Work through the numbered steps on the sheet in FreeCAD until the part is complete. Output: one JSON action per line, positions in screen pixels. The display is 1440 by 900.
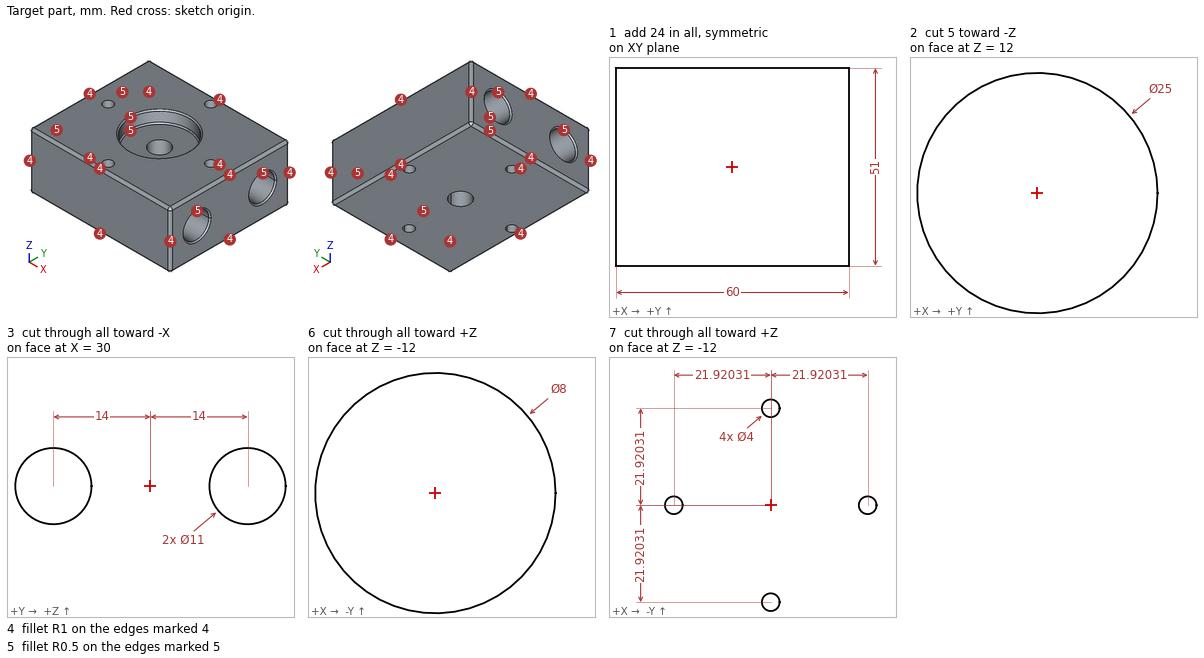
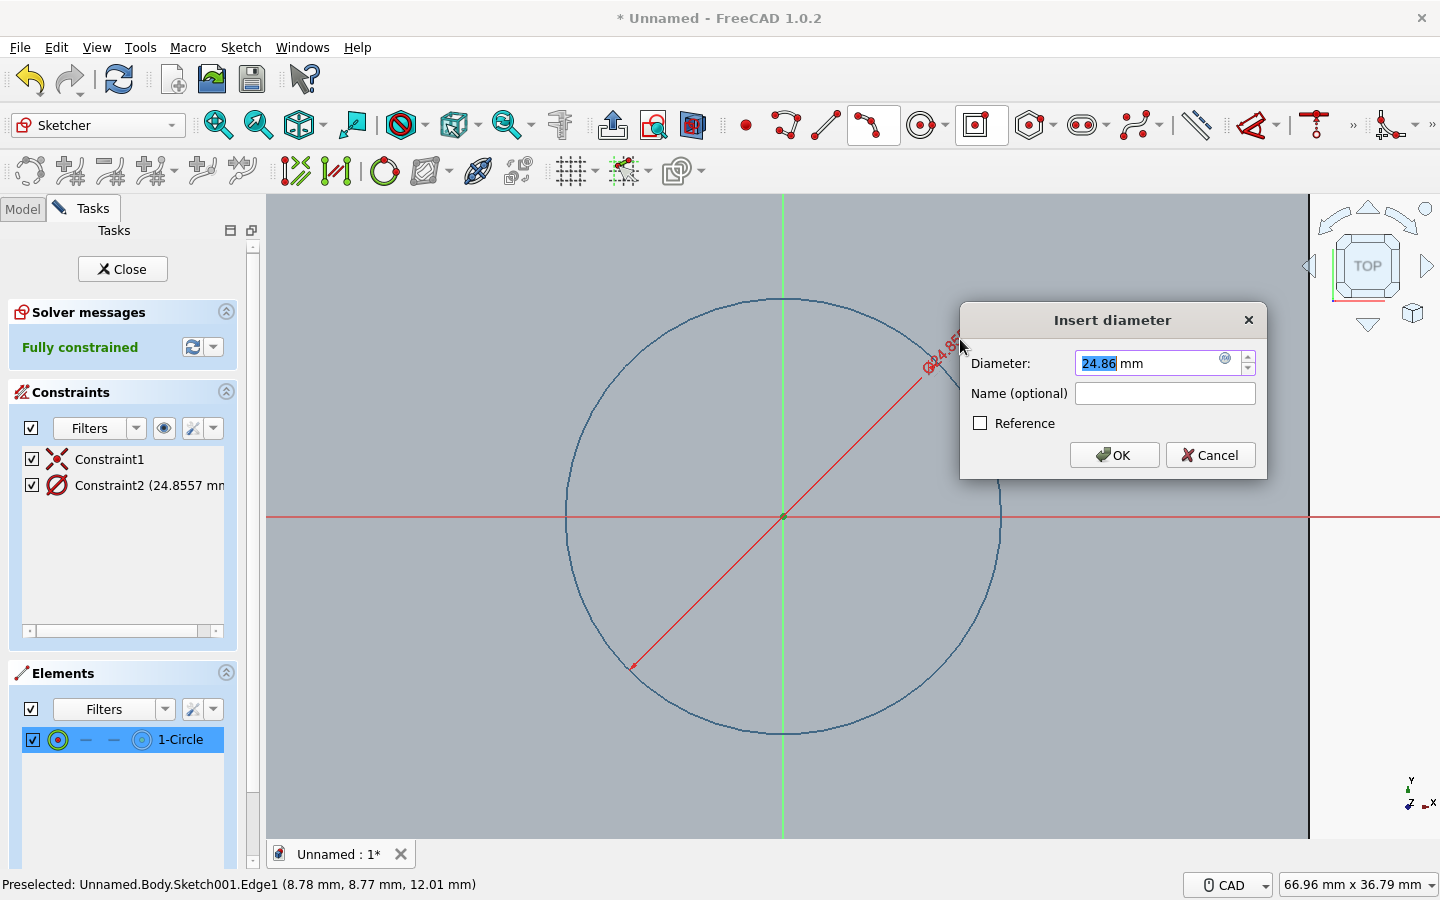
{"action": "type", "text": "25"}
{"action": "key", "text": "Return"}
{"action": "key", "text": "Escape"}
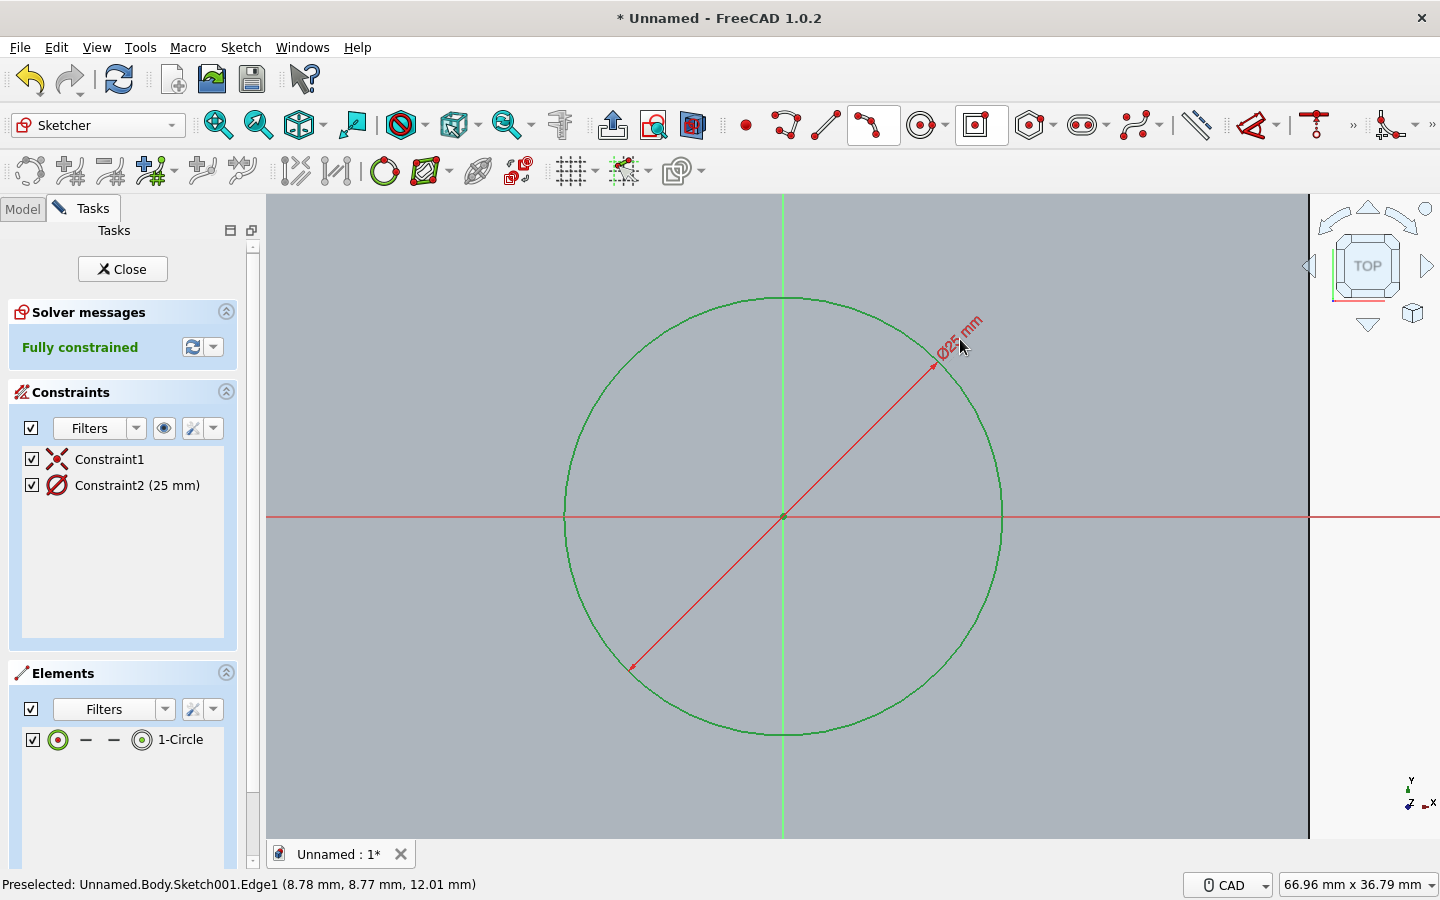
{"action": "left_click", "coordinate": [123, 269]}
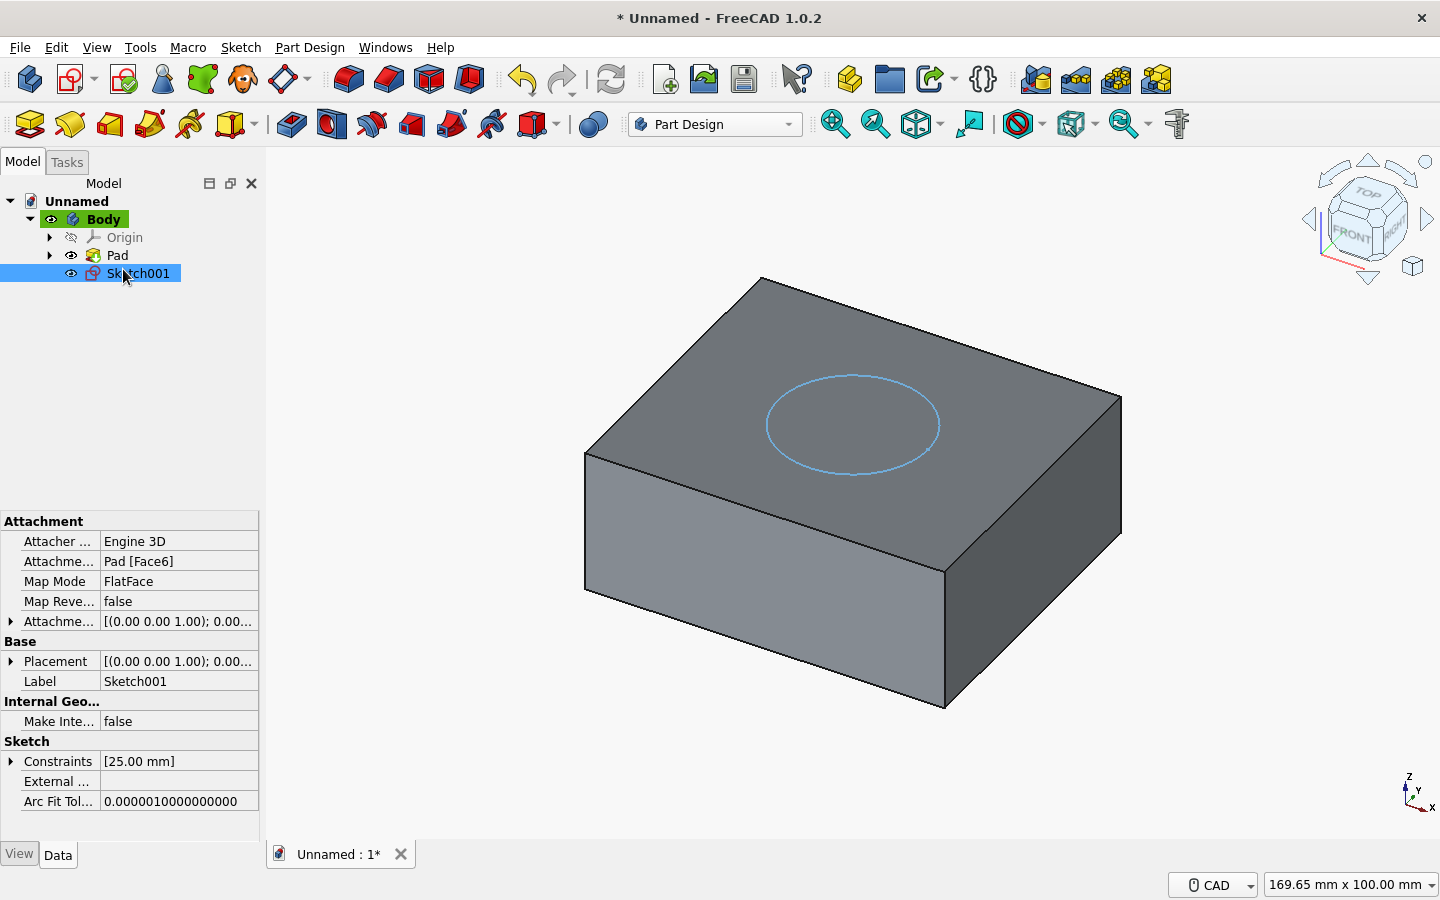
{"action": "left_click", "coordinate": [292, 124]}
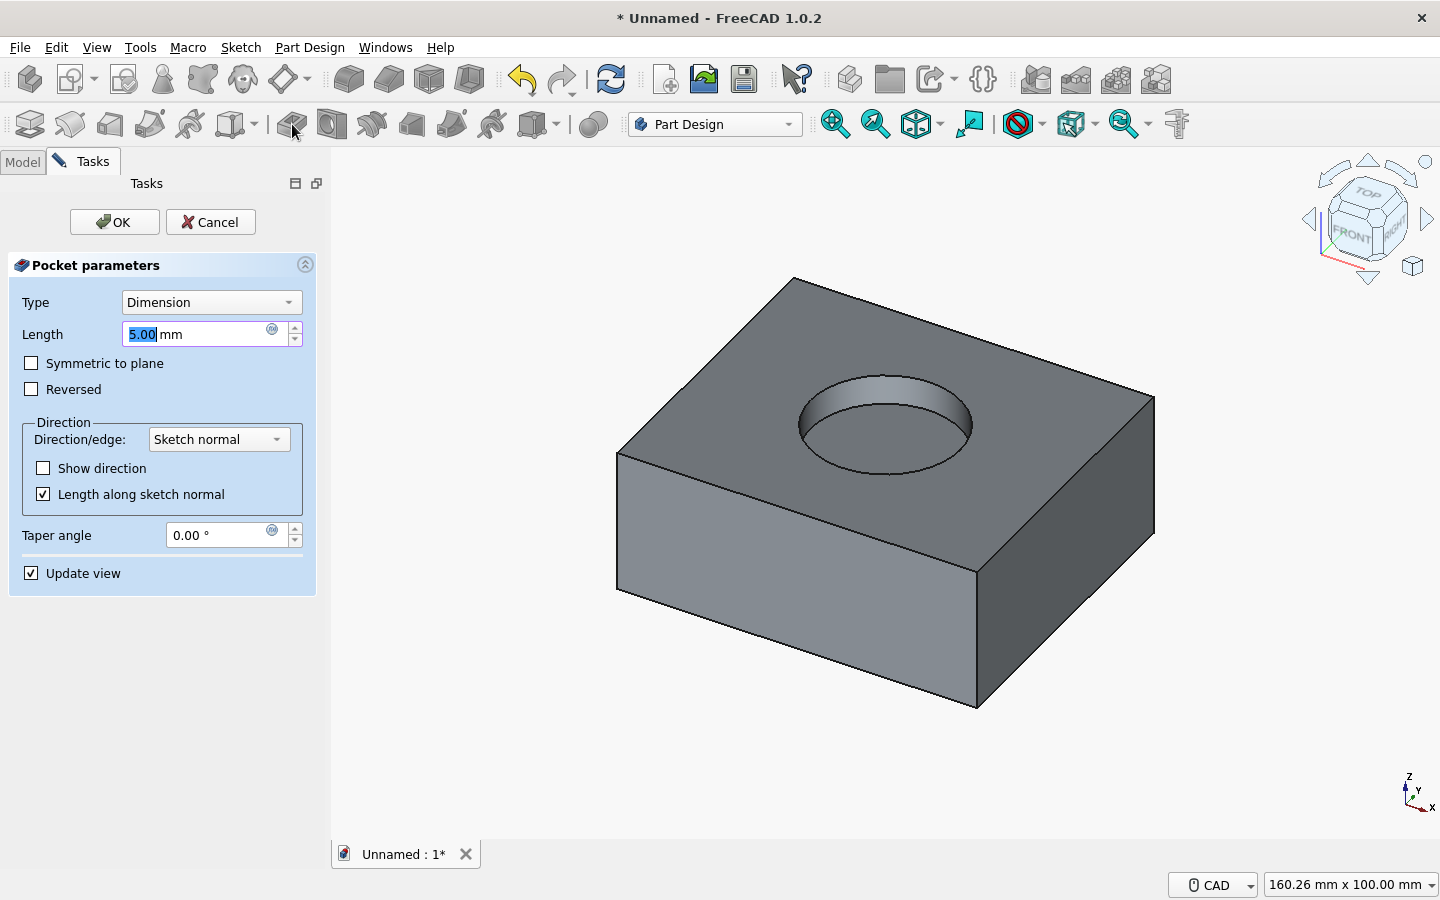
{"action": "type", "text": "5"}
{"action": "key", "text": "Tab"}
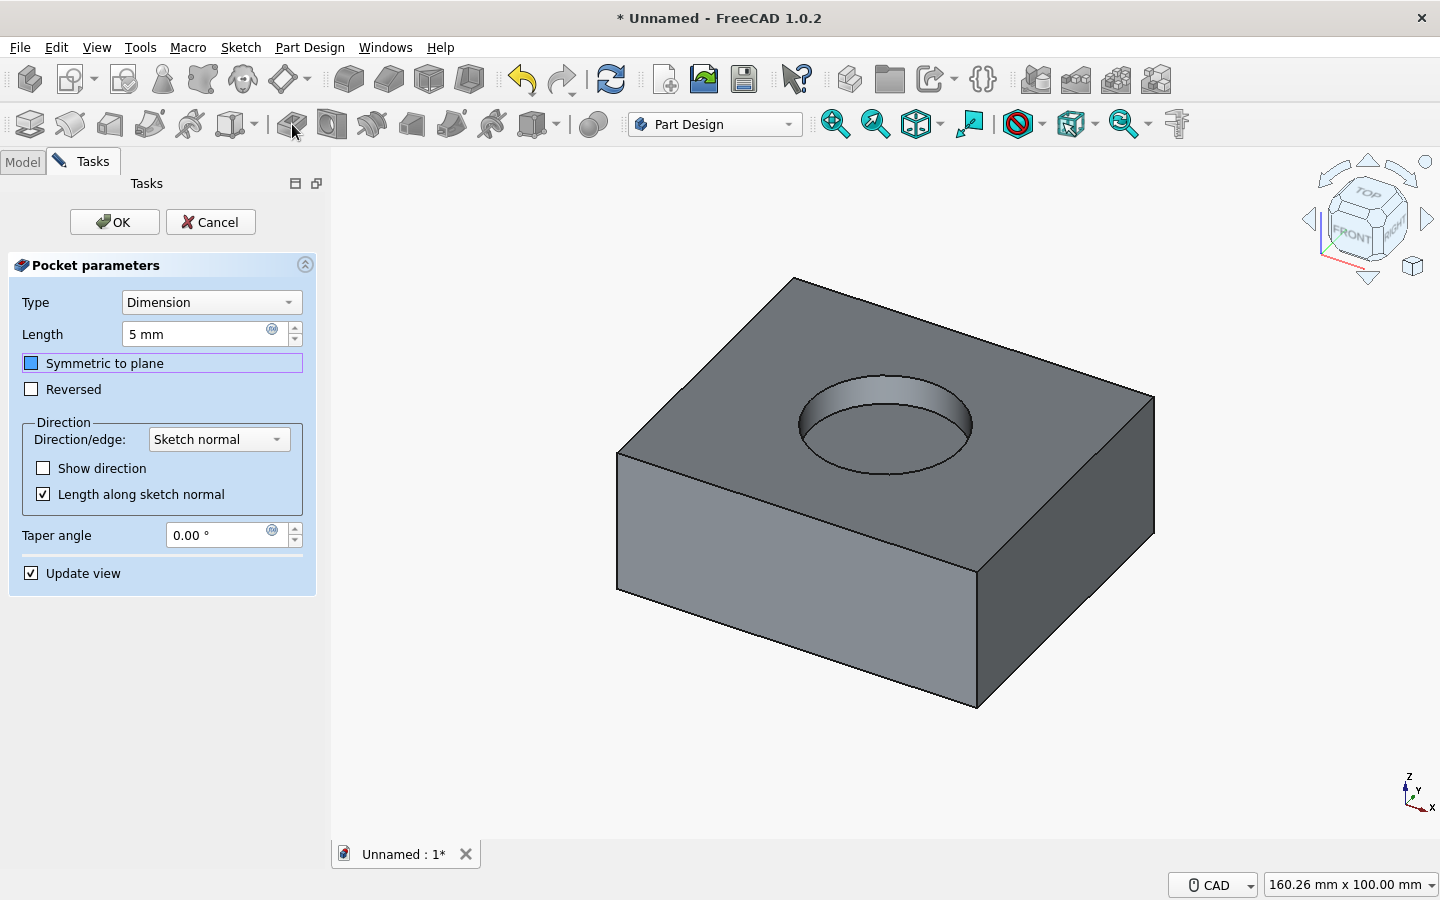
{"action": "left_click", "coordinate": [115, 222]}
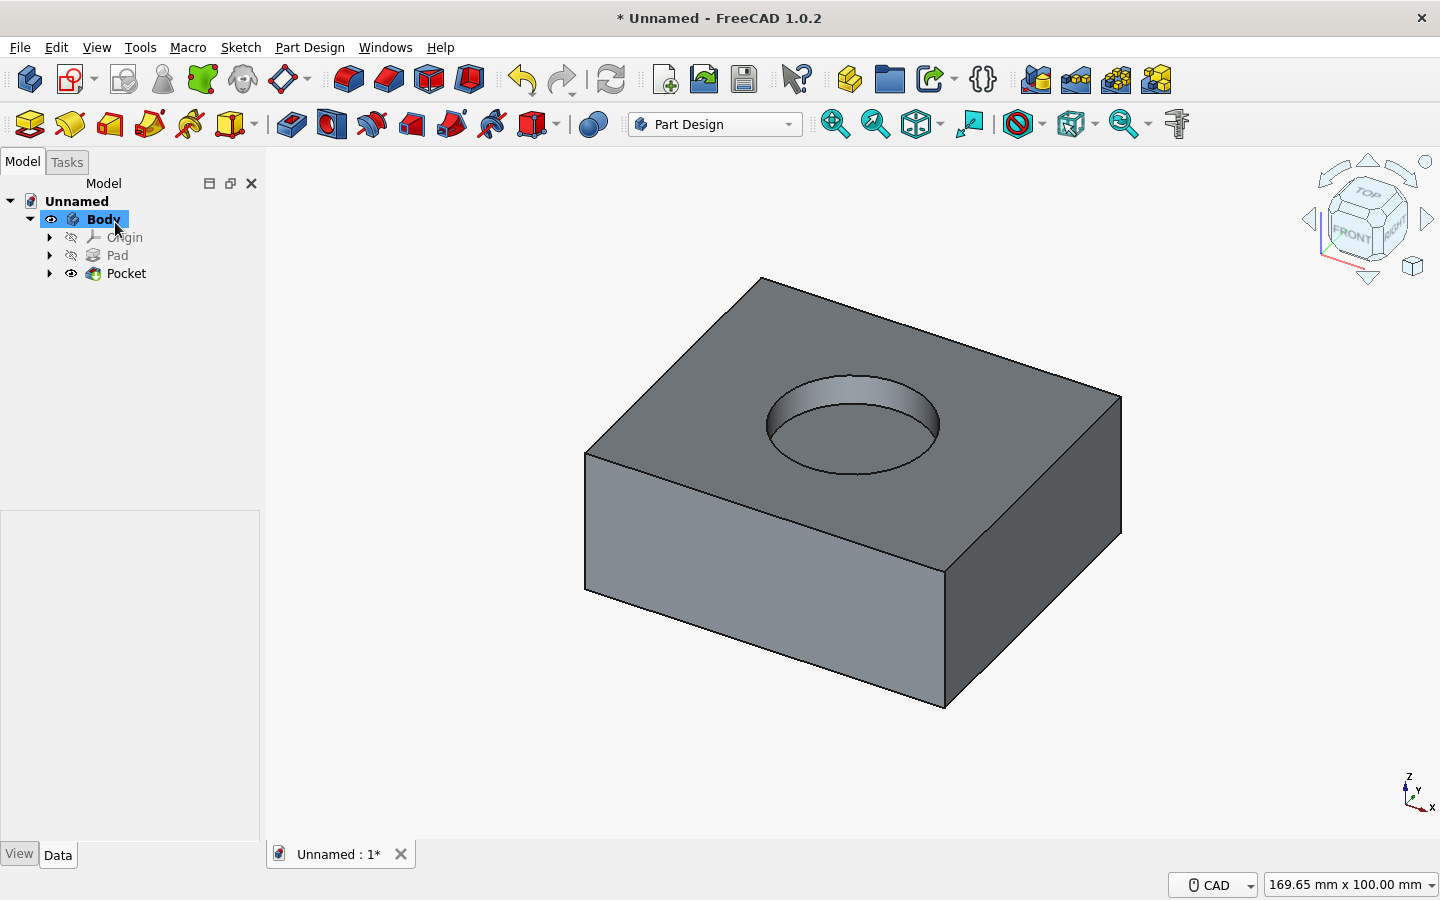
{"action": "left_click", "coordinate": [1058, 526]}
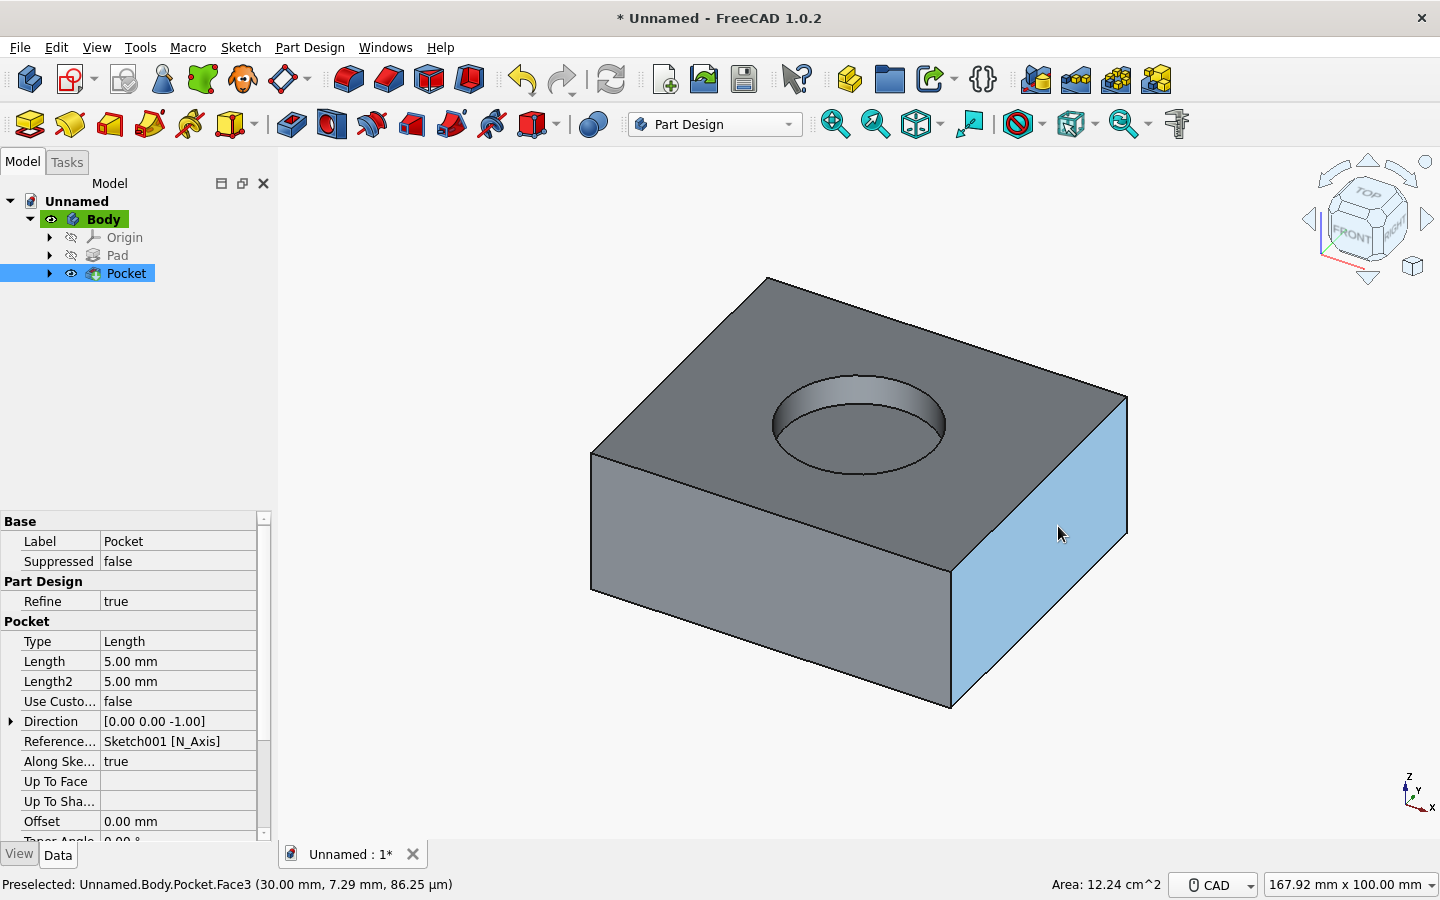
{"action": "left_click", "coordinate": [70, 80]}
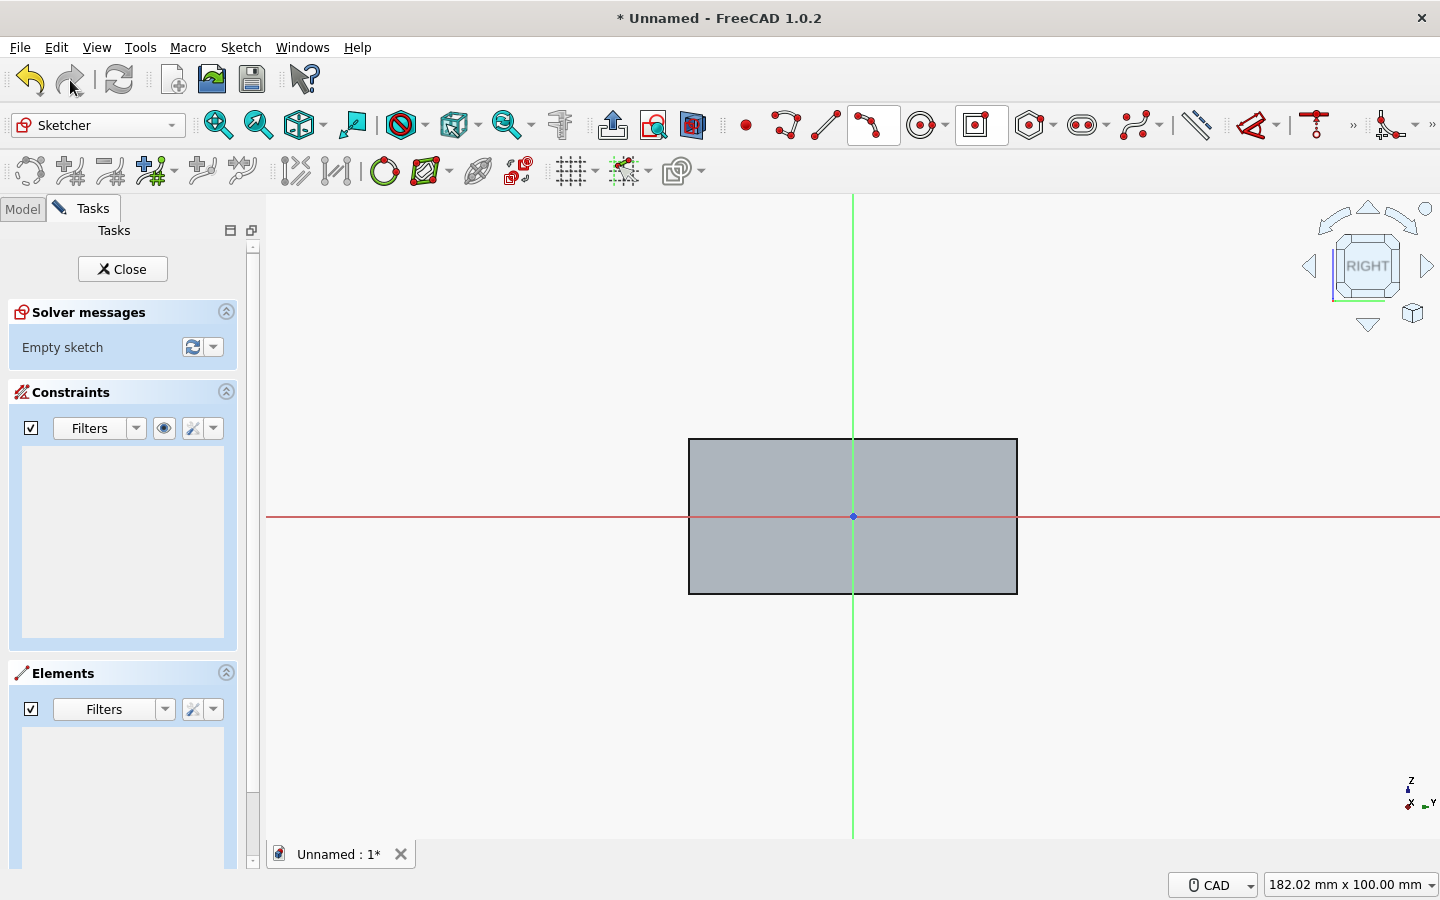
{"action": "scroll", "coordinate": [893, 516], "scroll_direction": "up", "scroll_amount": 5}